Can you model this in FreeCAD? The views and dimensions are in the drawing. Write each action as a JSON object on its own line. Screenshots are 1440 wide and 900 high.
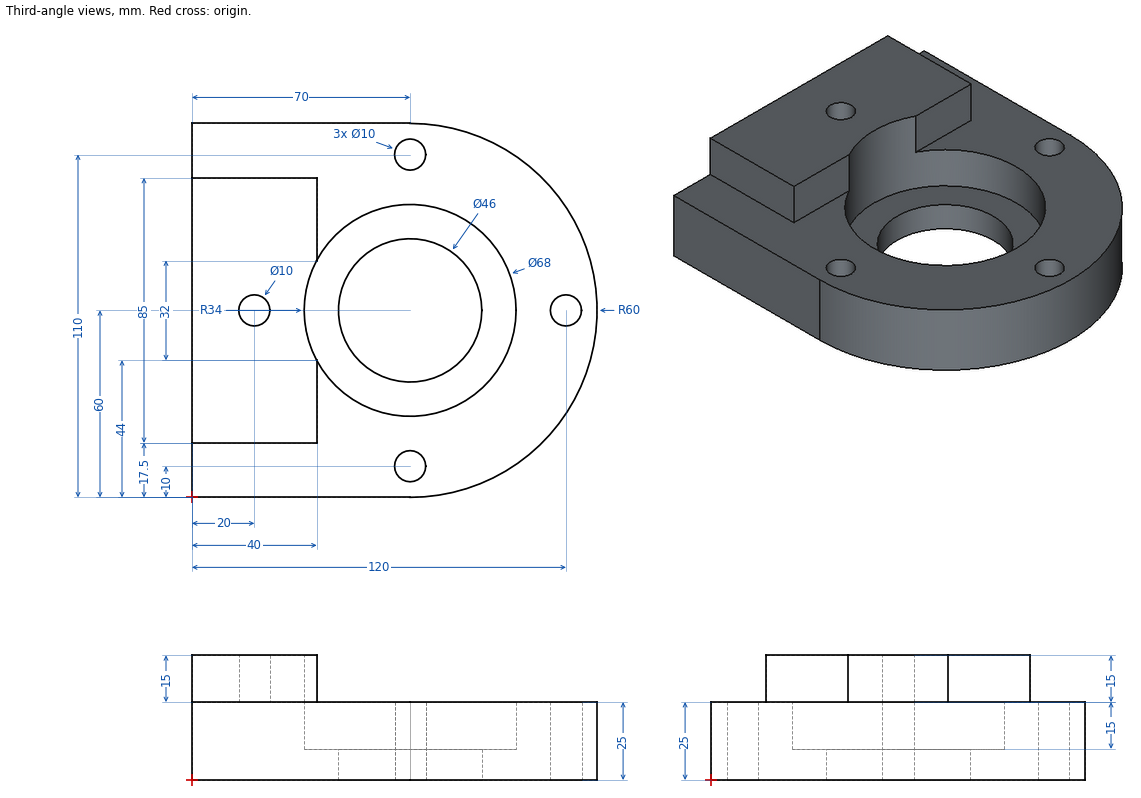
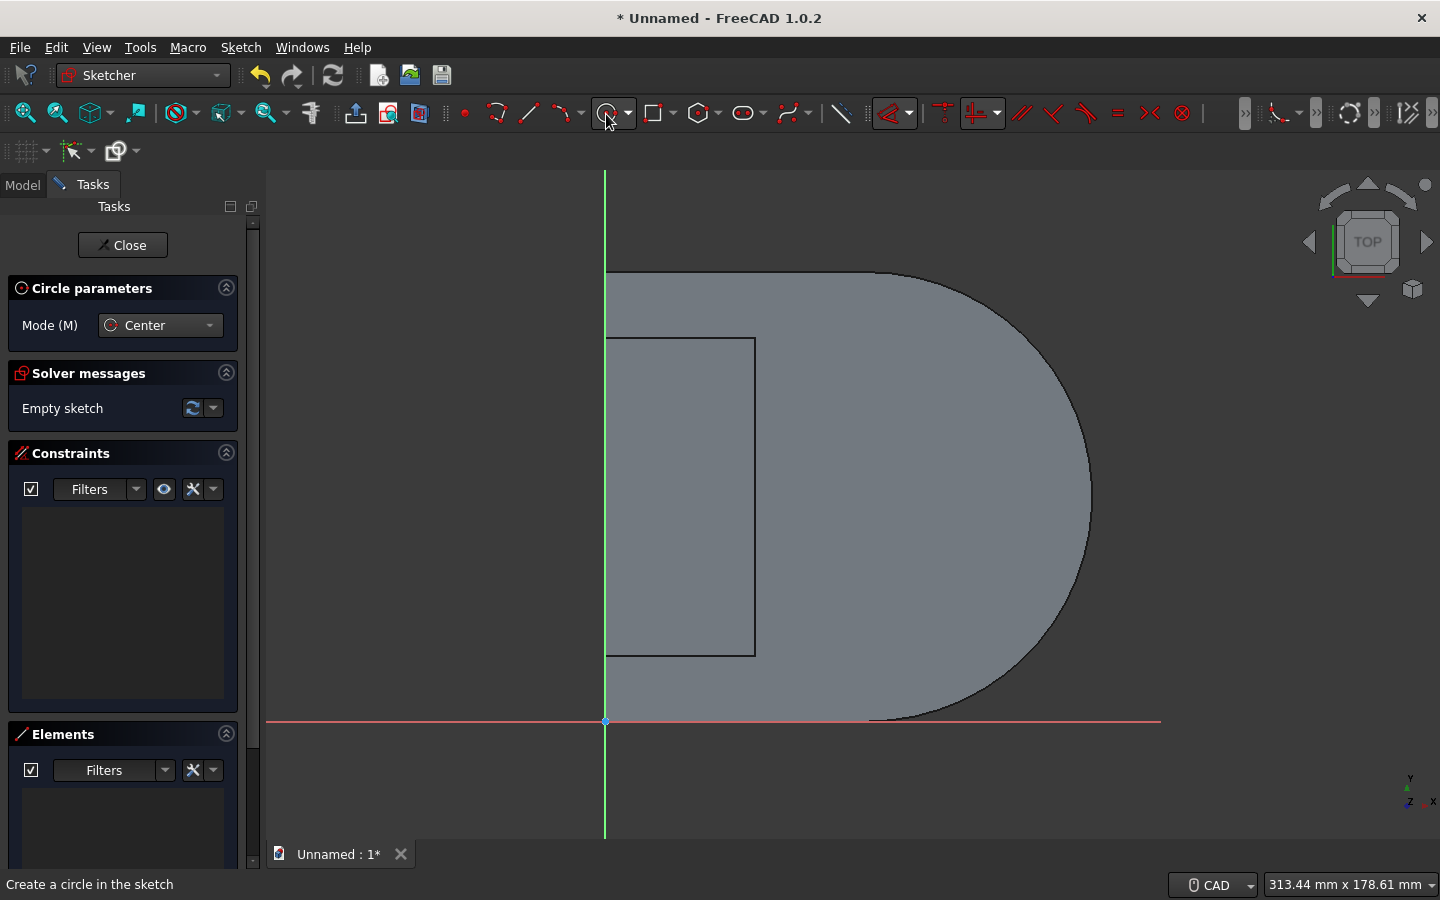
{"action": "left_click", "coordinate": [867, 497]}
{"action": "left_click", "coordinate": [958, 407]}
{"action": "key", "text": "Escape"}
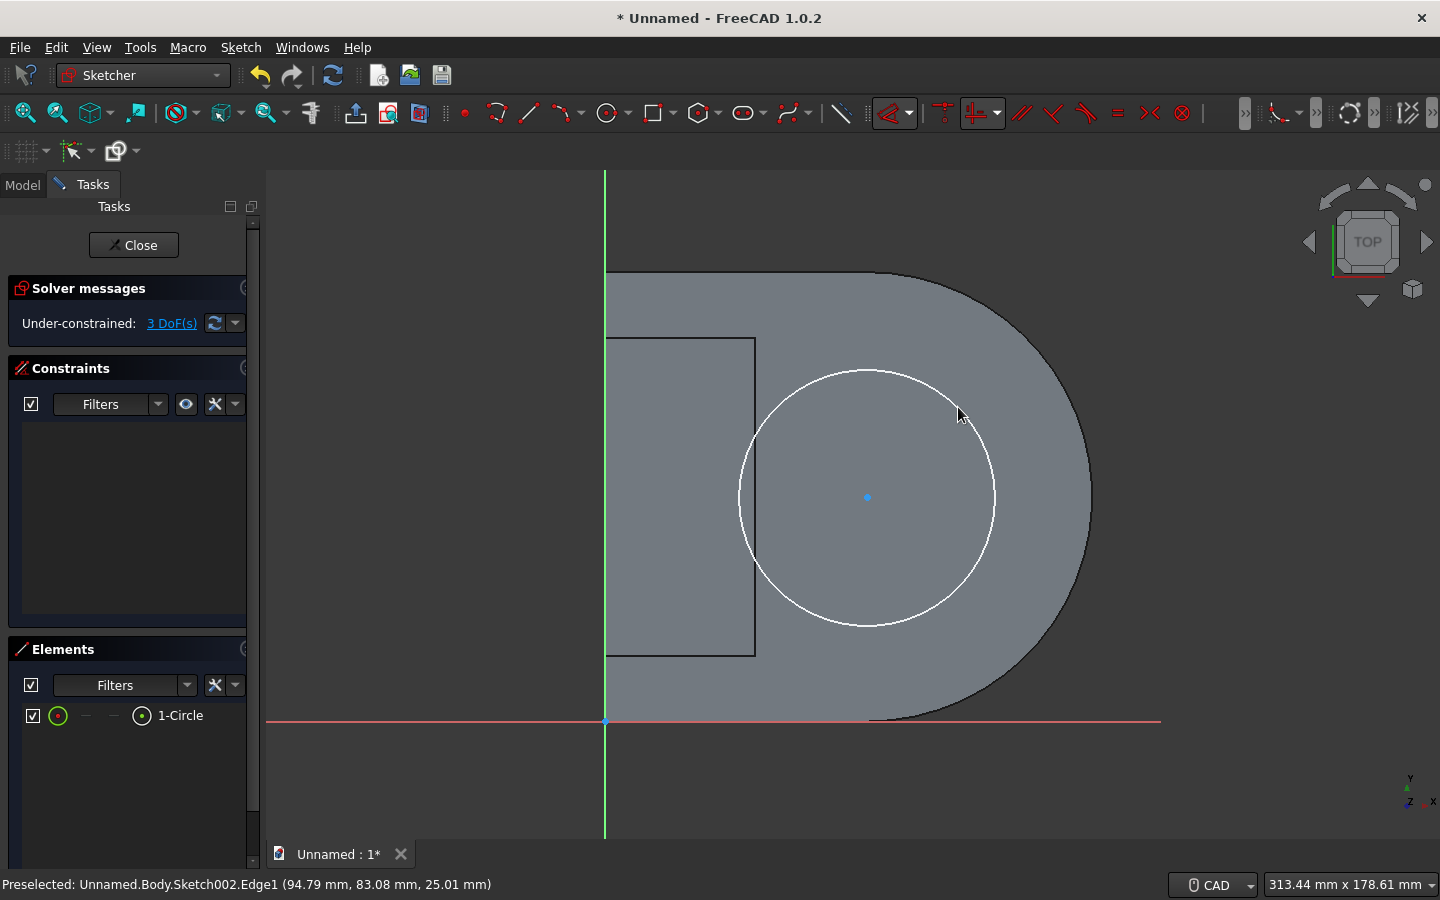
{"action": "left_click", "coordinate": [957, 407]}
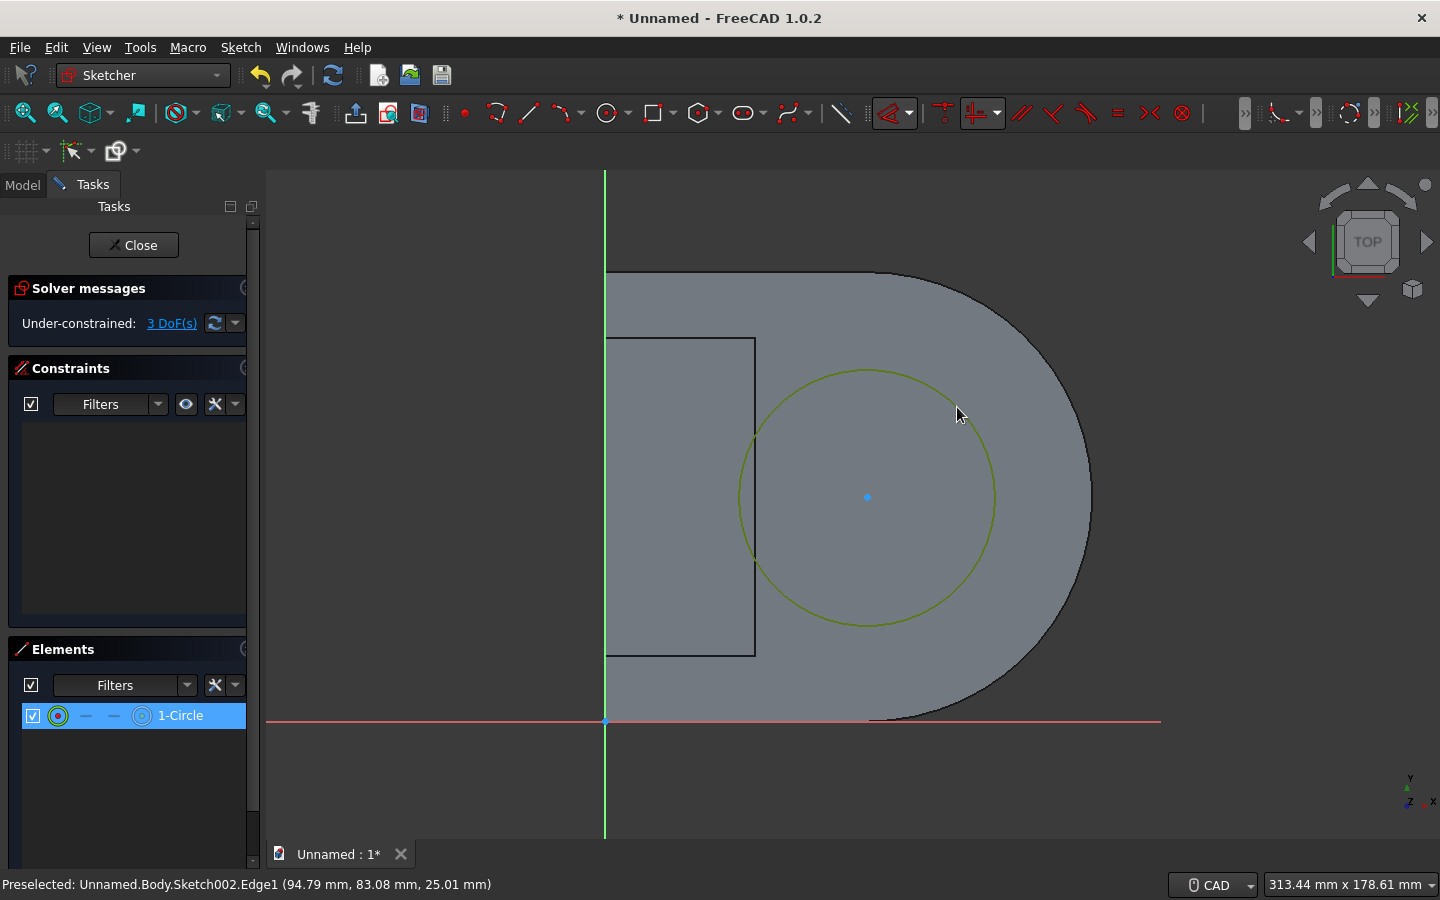
{"action": "key", "text": "k o"}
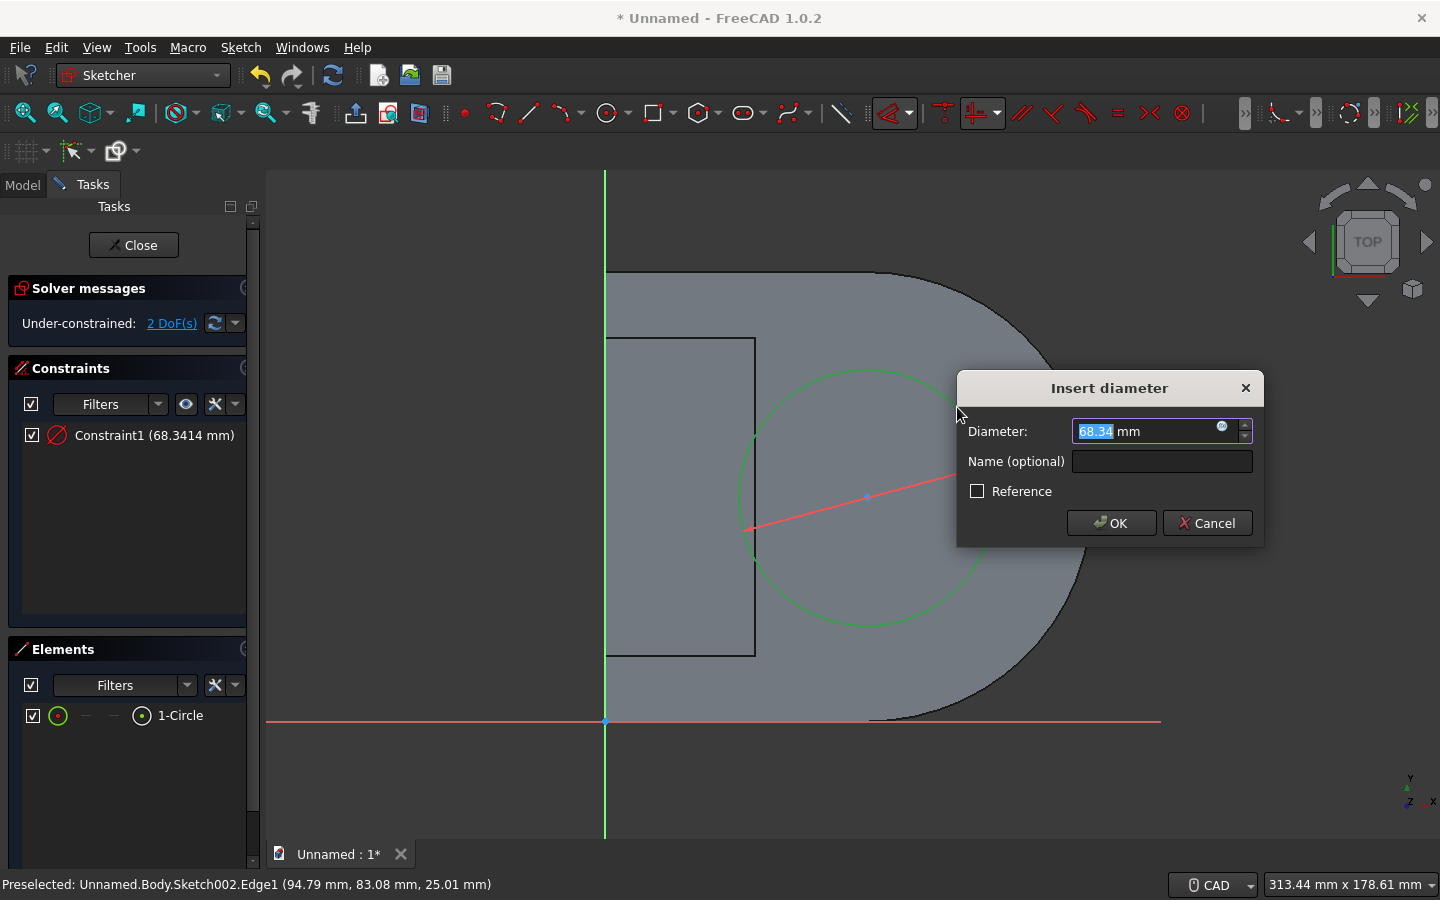
{"action": "type", "text": "68"}
{"action": "key", "text": "Return"}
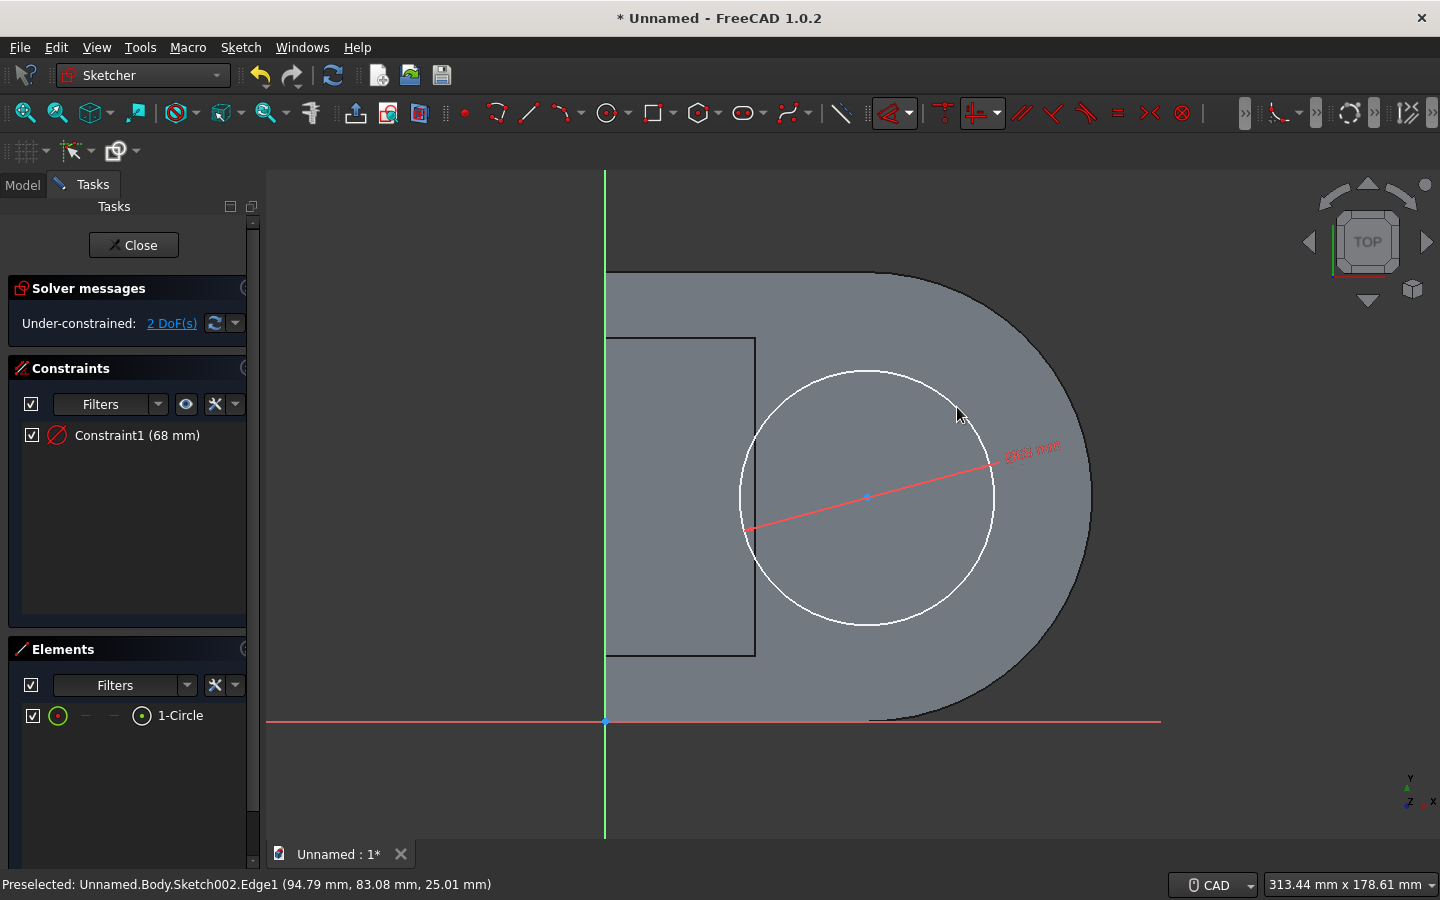
{"action": "left_click", "coordinate": [867, 498]}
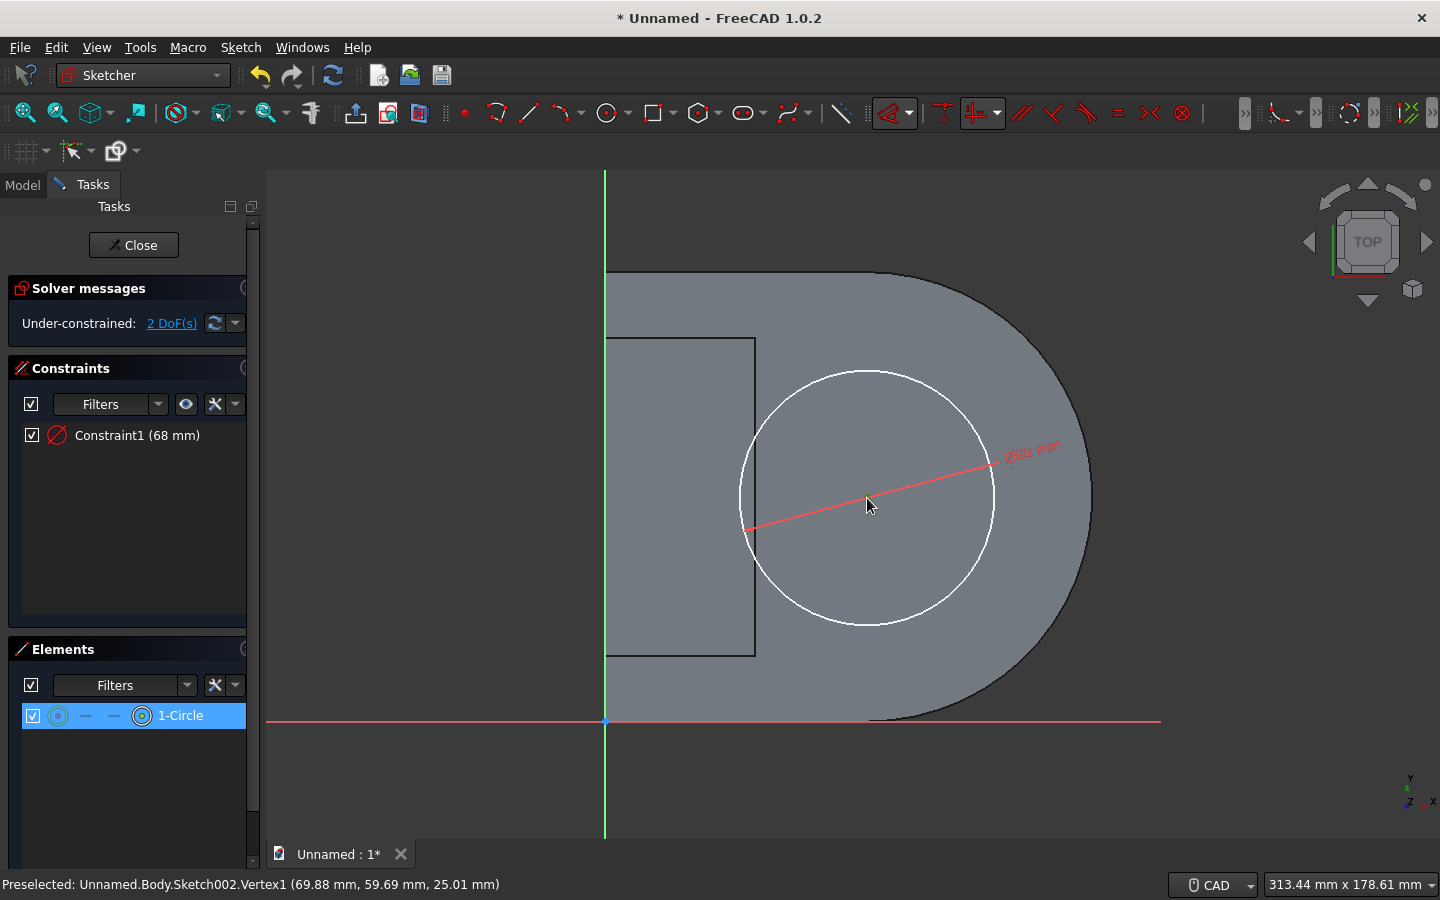
{"action": "left_click", "coordinate": [912, 114]}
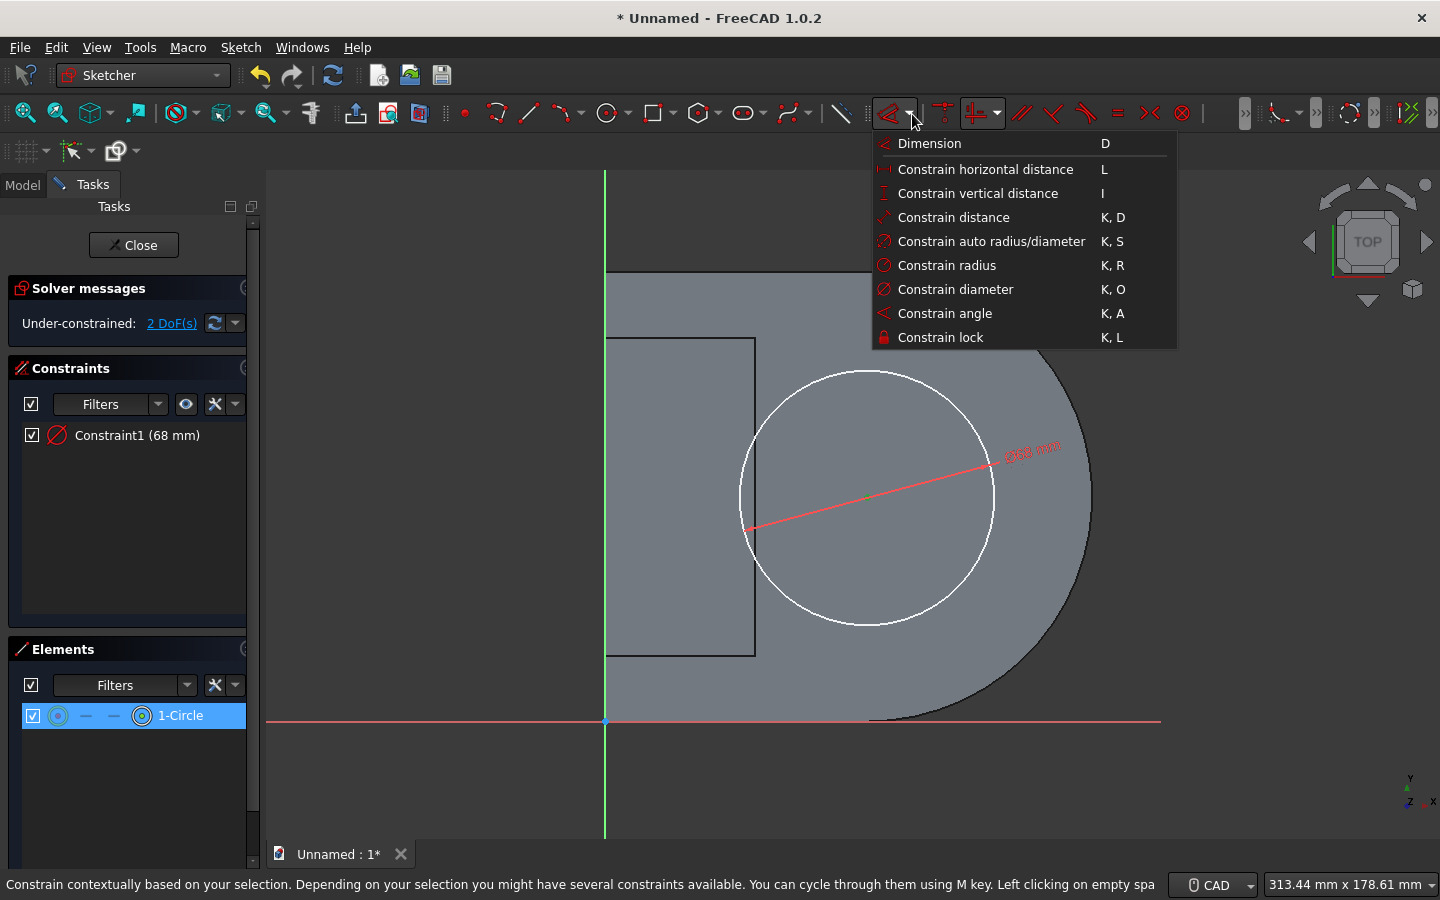
{"action": "left_click", "coordinate": [1025, 169]}